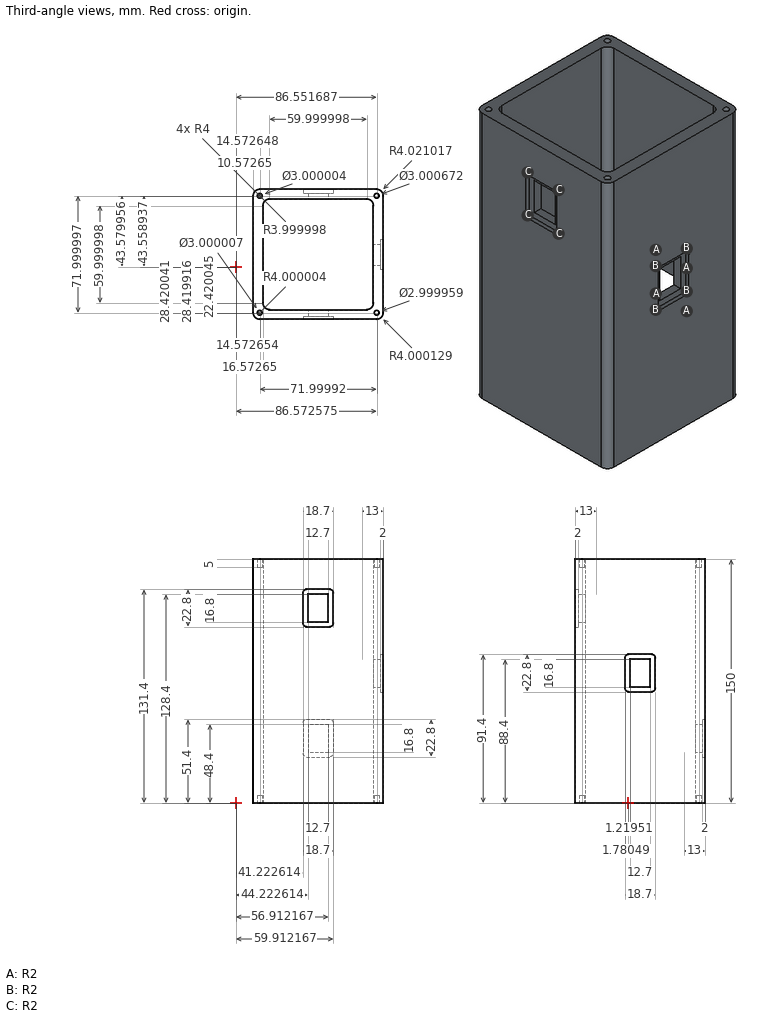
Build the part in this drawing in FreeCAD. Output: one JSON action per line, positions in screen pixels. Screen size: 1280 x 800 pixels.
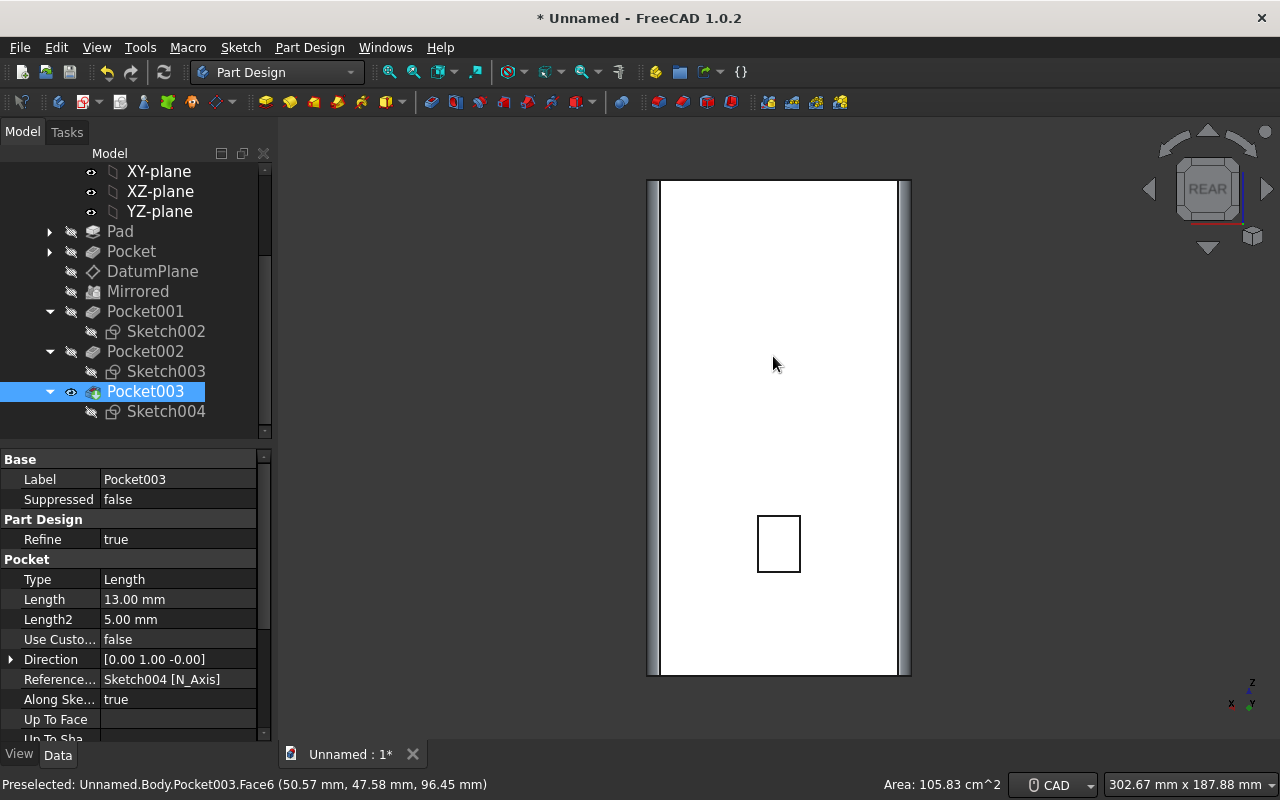
{"action": "left_click", "coordinate": [84, 102]}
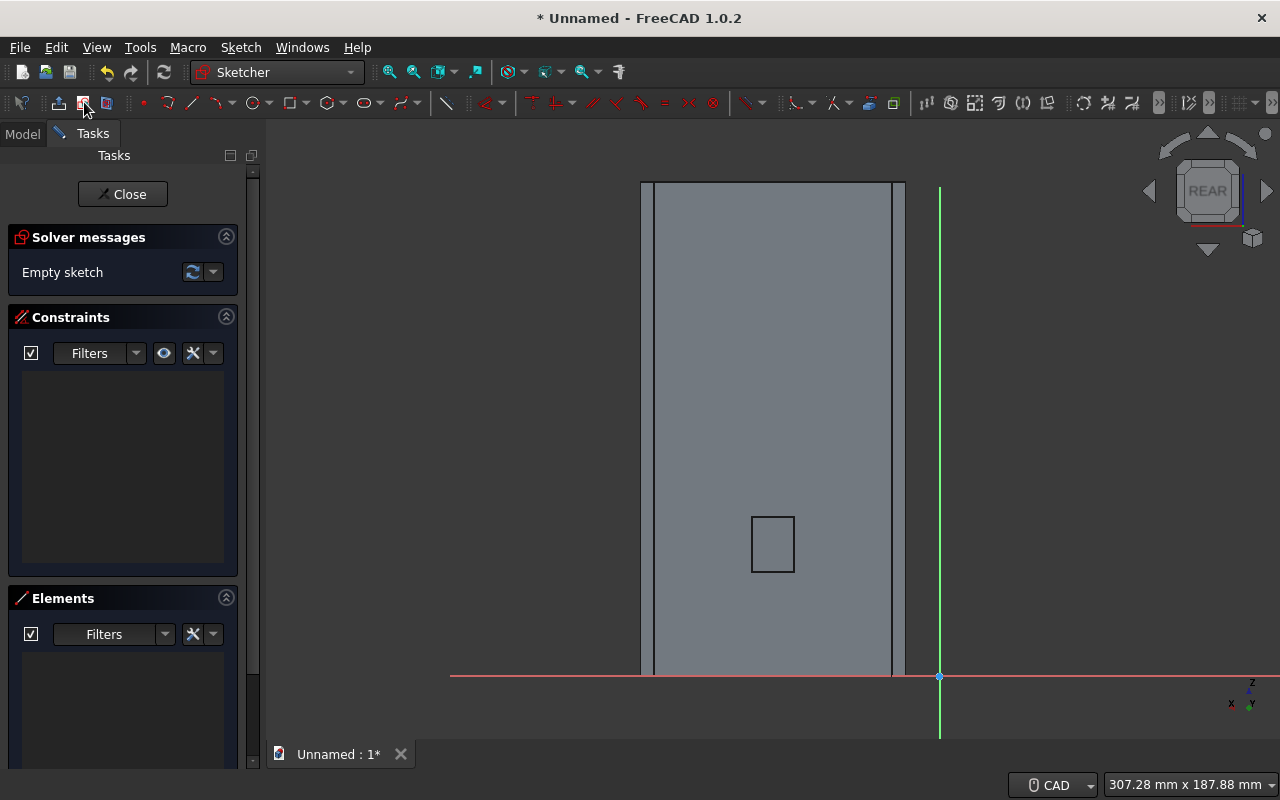
{"action": "scroll", "coordinate": [790, 574], "scroll_direction": "up", "scroll_amount": 8}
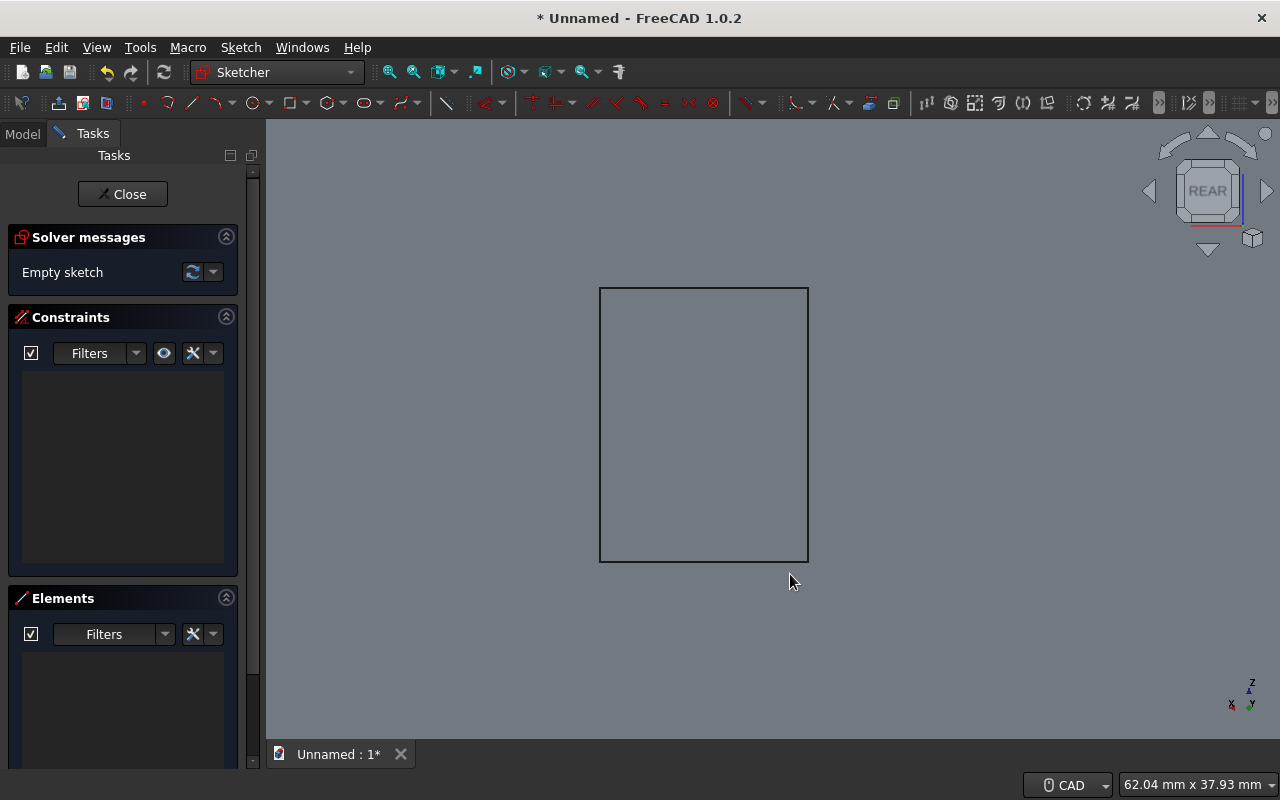
{"action": "left_click", "coordinate": [290, 104]}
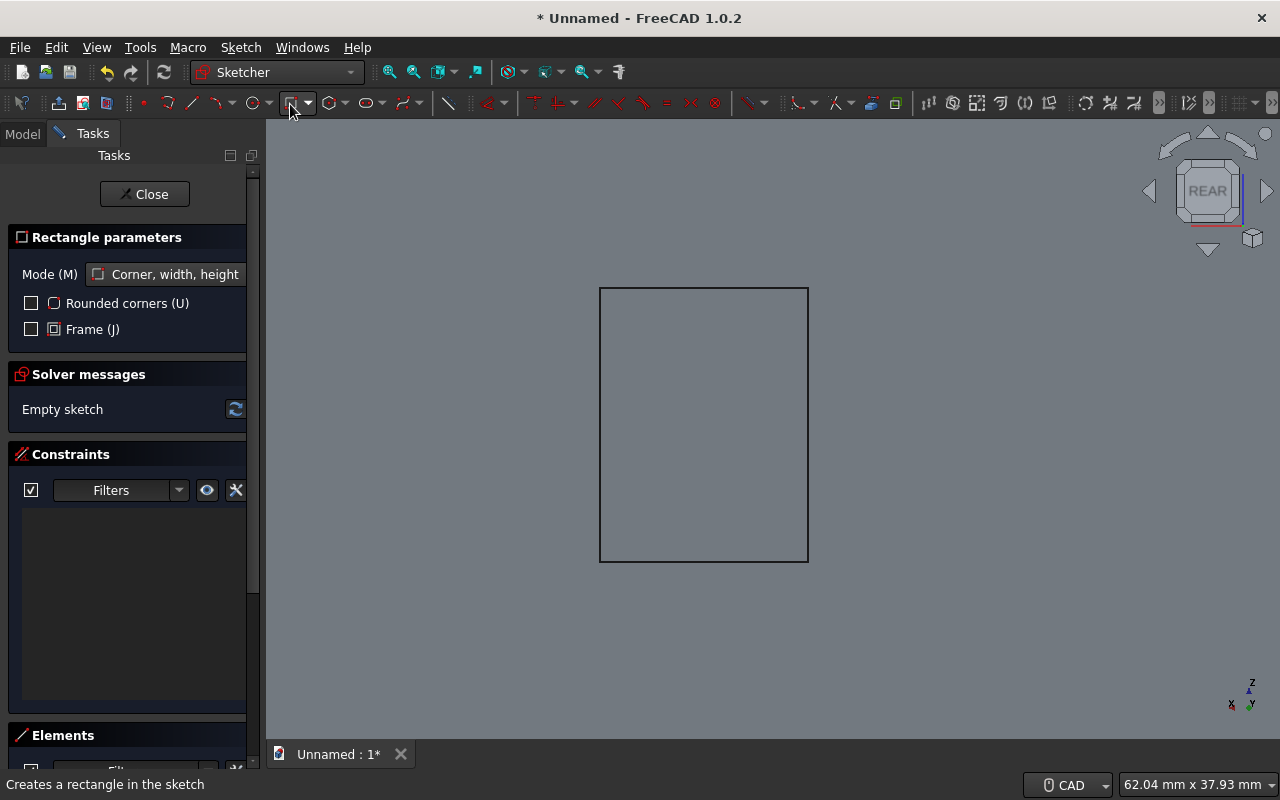
{"action": "left_click", "coordinate": [551, 239]}
{"action": "left_click", "coordinate": [857, 611]}
{"action": "key", "text": "Escape"}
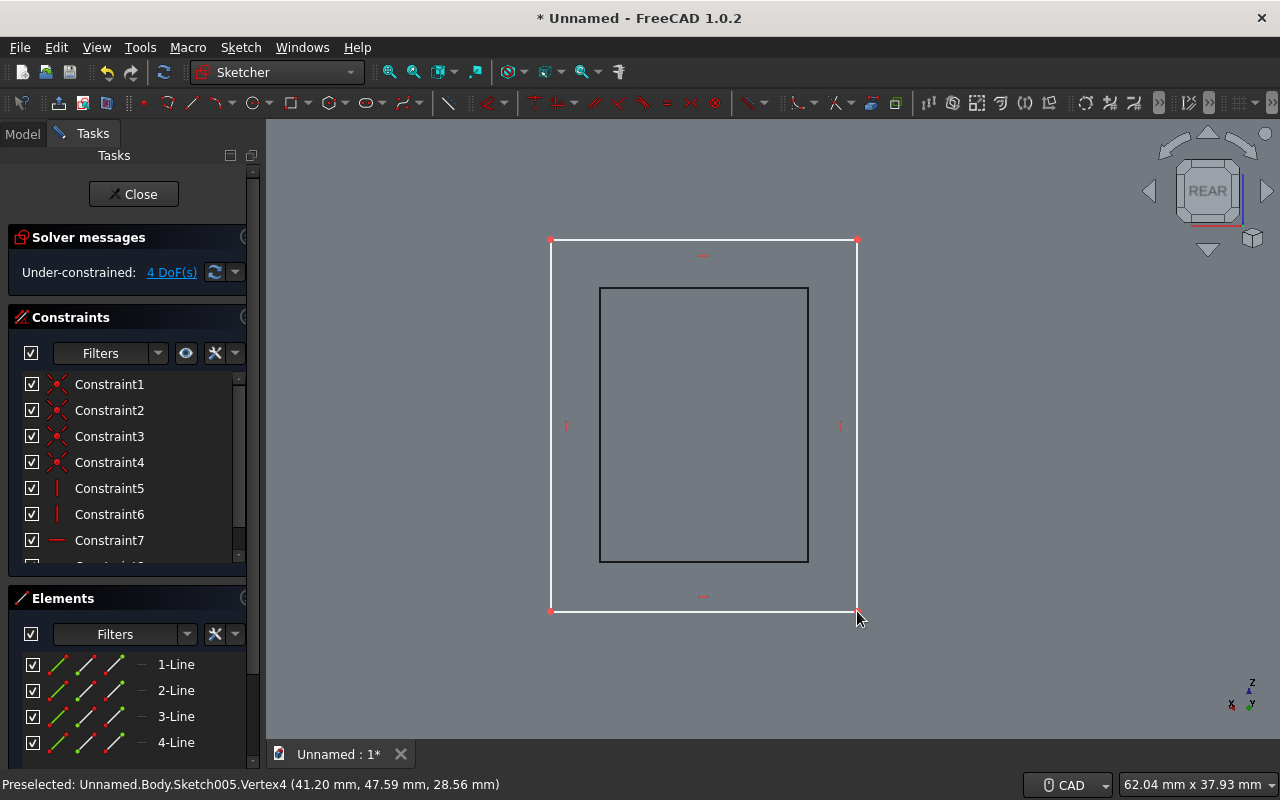
{"action": "left_click", "coordinate": [488, 104]}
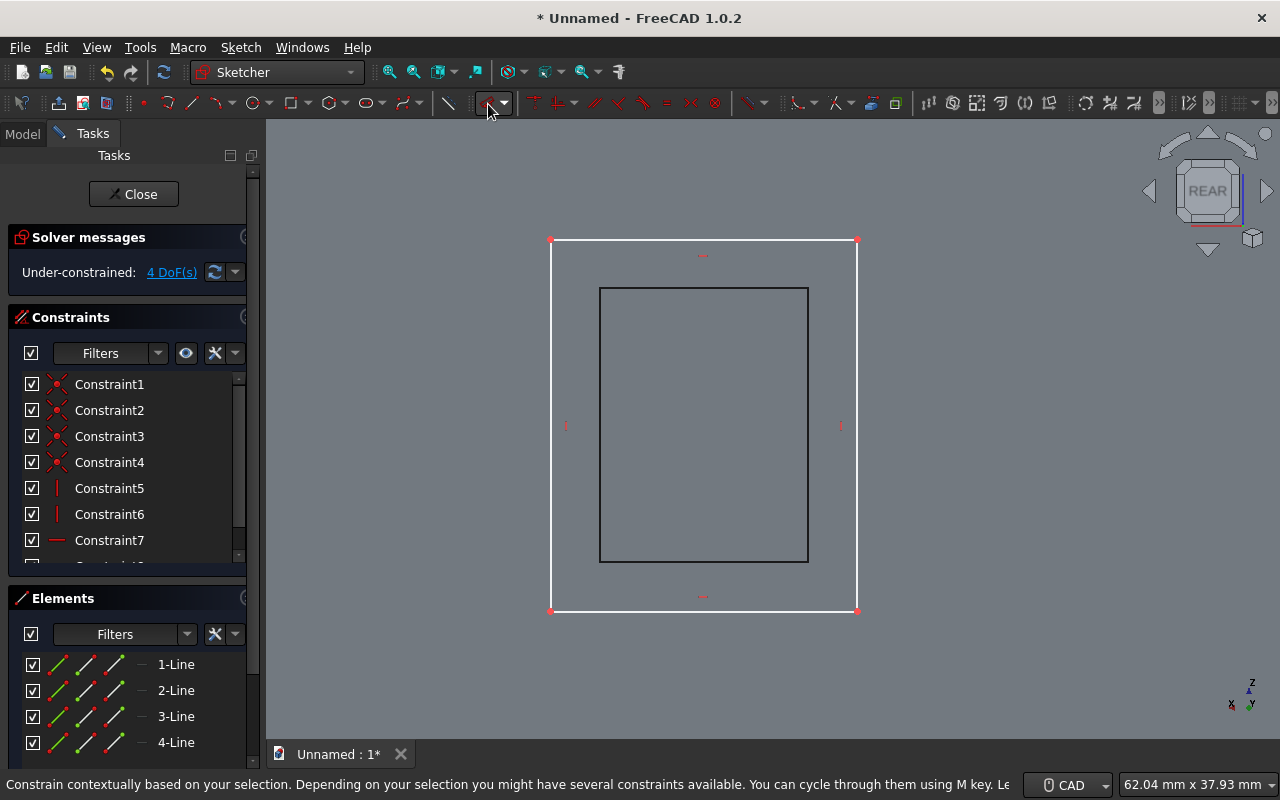
{"action": "left_click", "coordinate": [551, 352]}
{"action": "left_click", "coordinate": [517, 426]}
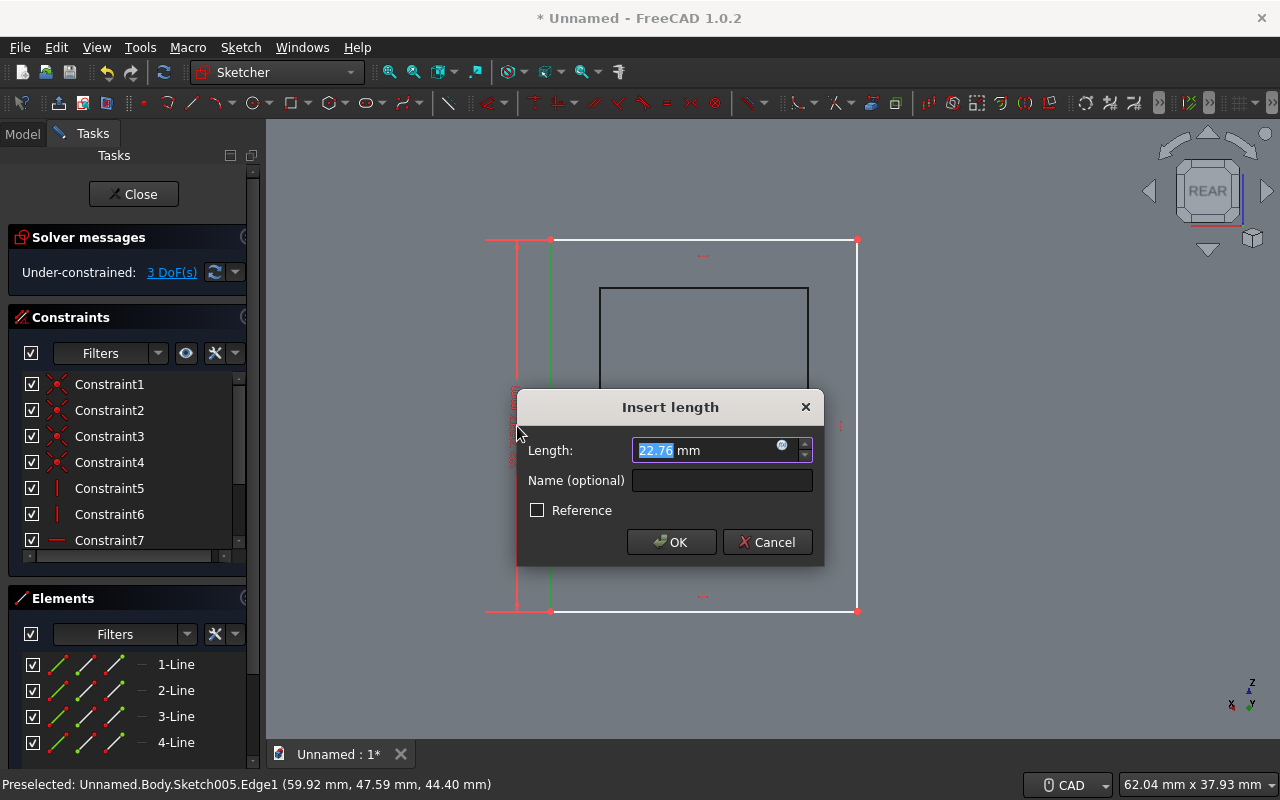
{"action": "type", "text": "22.8"}
{"action": "key", "text": "Return"}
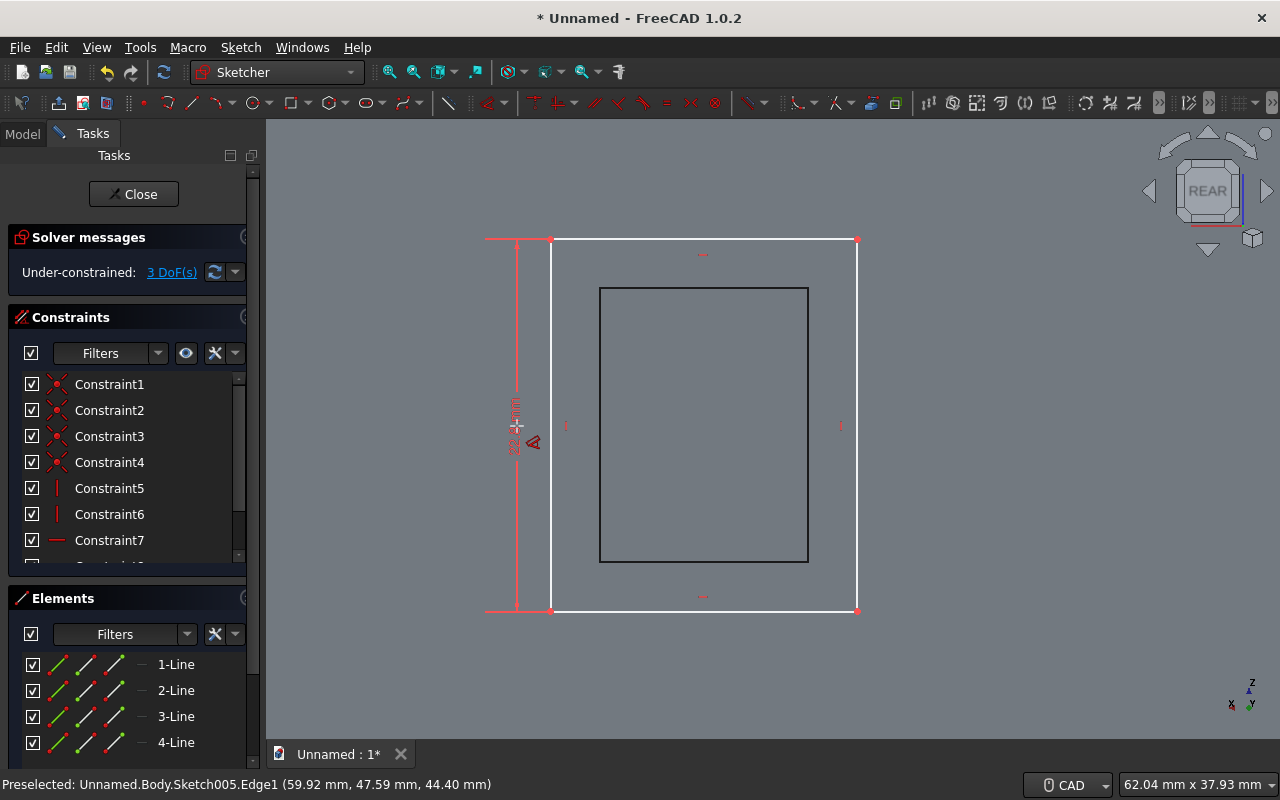
{"action": "left_click", "coordinate": [643, 612]}
{"action": "left_click", "coordinate": [704, 646]}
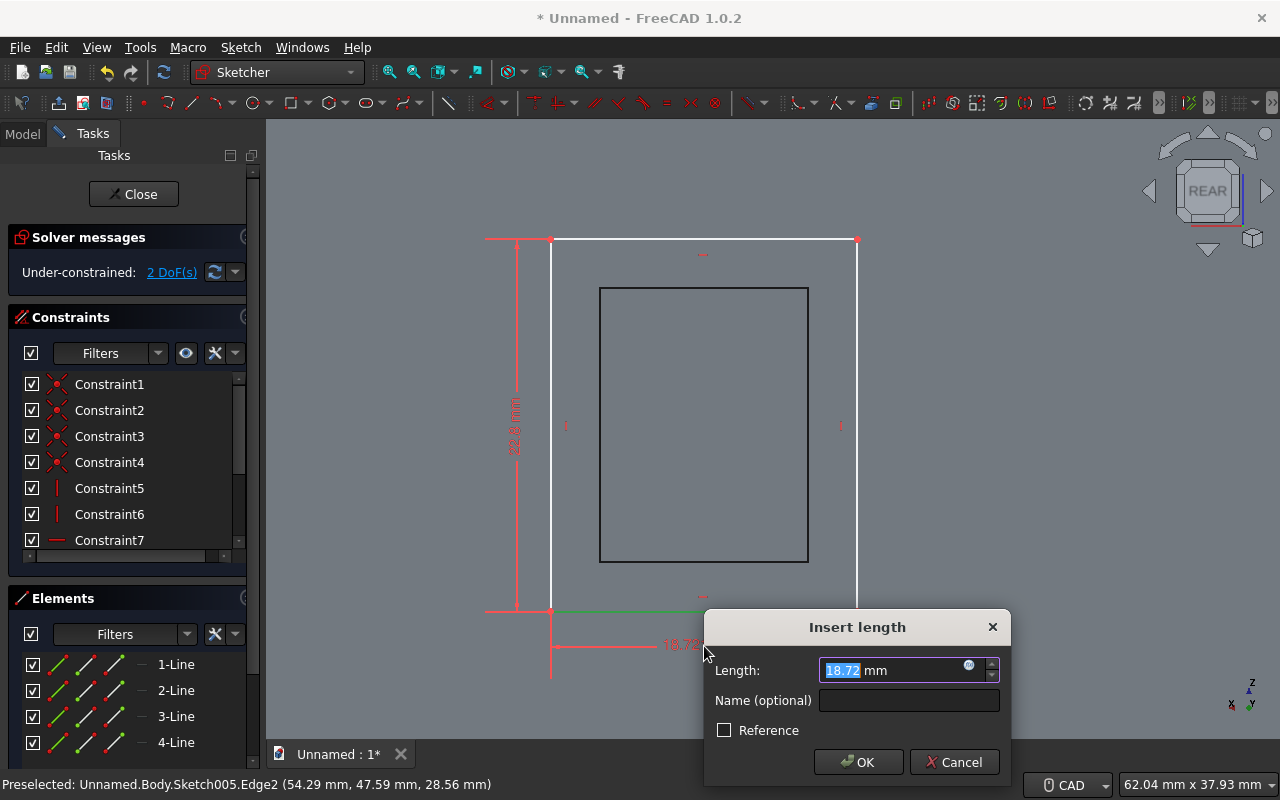
{"action": "type", "text": "18.7"}
{"action": "key", "text": "Return"}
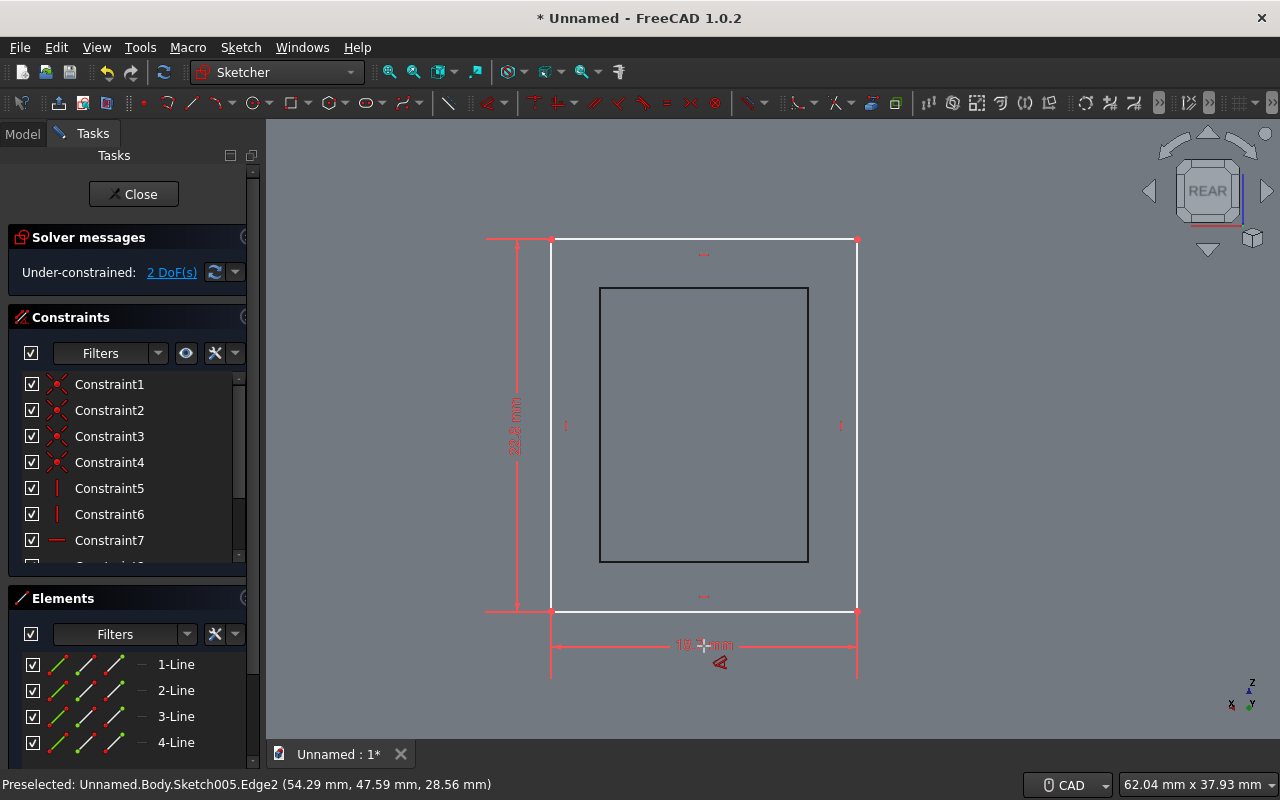
{"action": "left_click", "coordinate": [551, 239]}
{"action": "left_click", "coordinate": [517, 475]}